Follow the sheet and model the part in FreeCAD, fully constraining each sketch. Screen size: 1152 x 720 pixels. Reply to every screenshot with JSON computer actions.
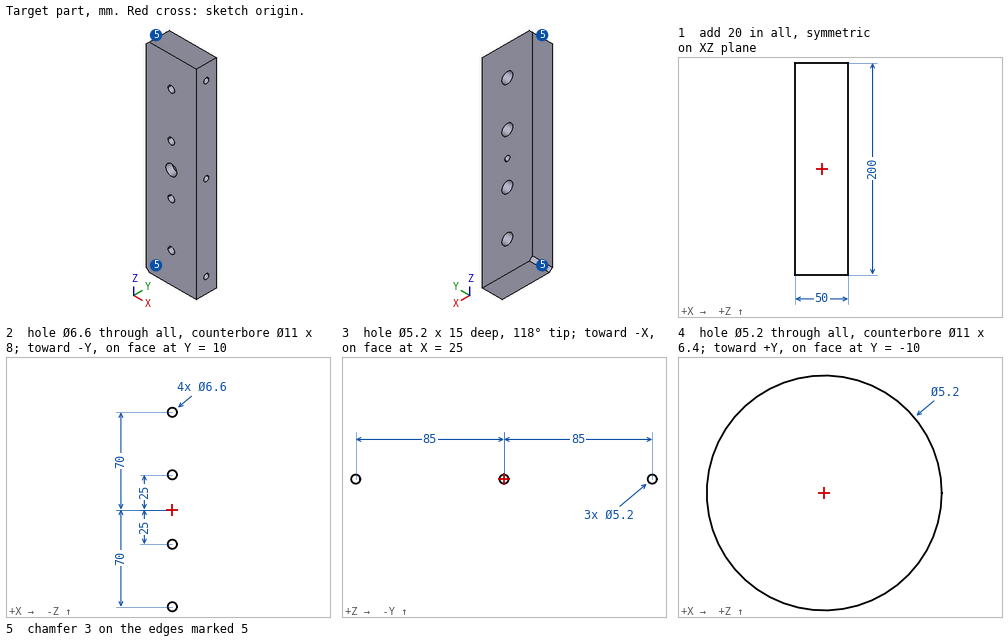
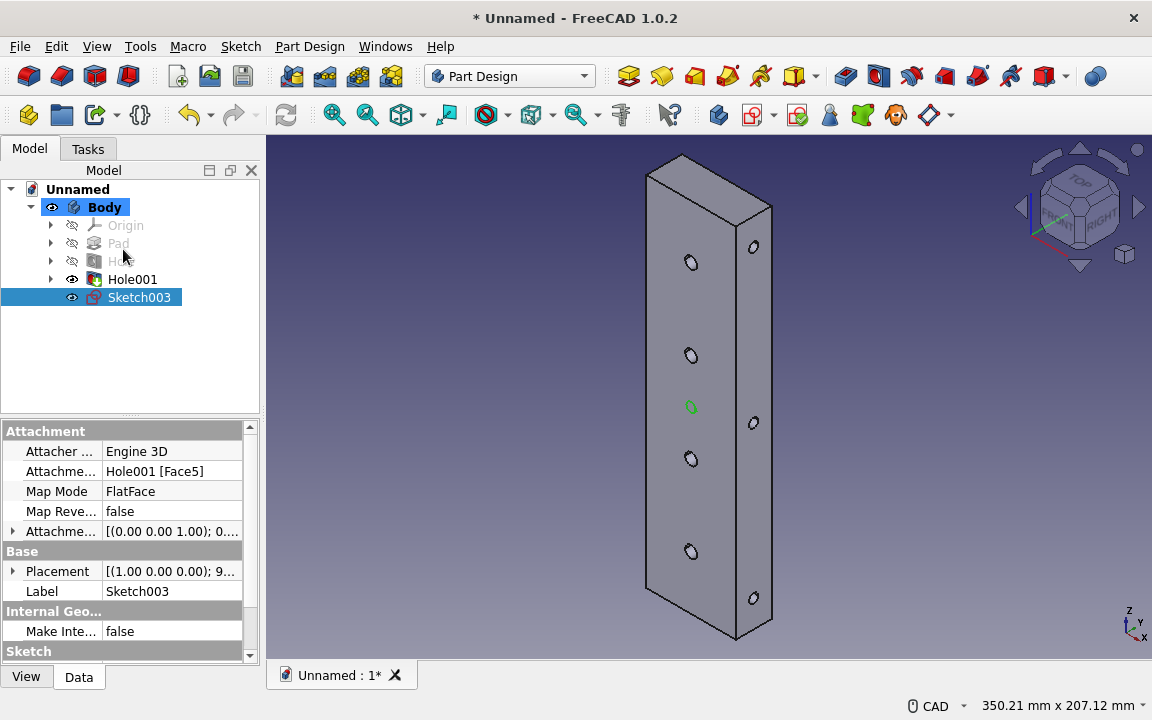
{"action": "left_click", "coordinate": [879, 76]}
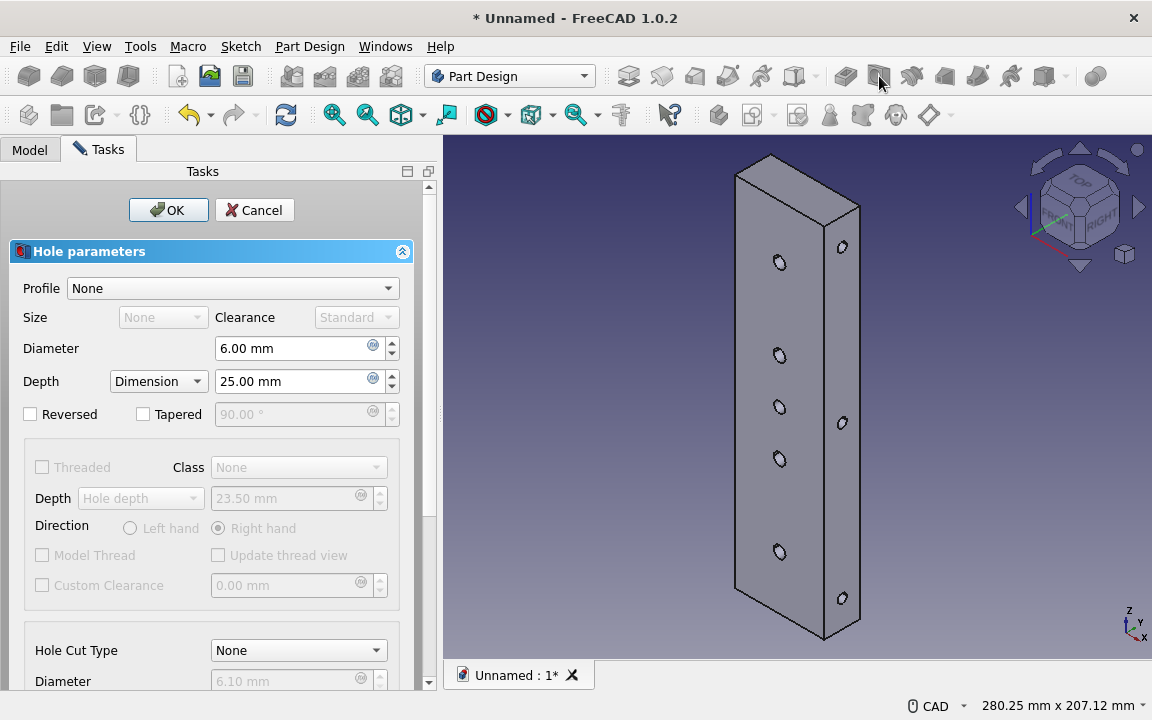
{"action": "triple_click", "coordinate": [300, 348]}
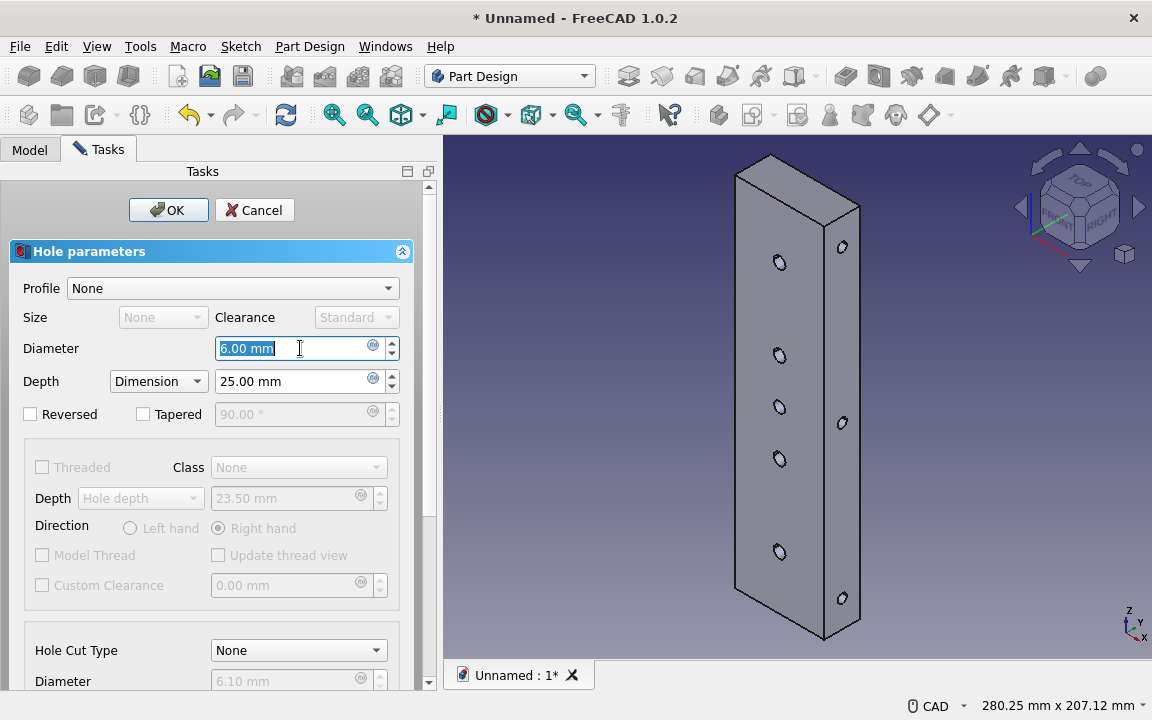
{"action": "type", "text": "5.2"}
{"action": "key", "text": "Tab"}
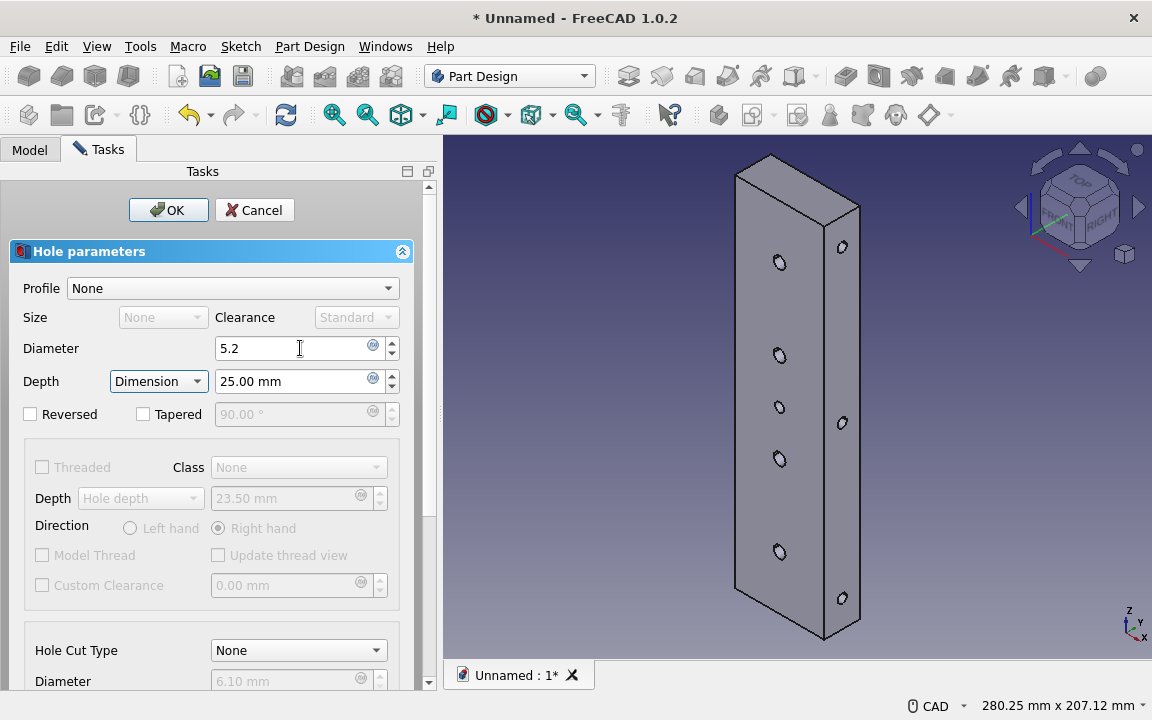
{"action": "left_click", "coordinate": [160, 382]}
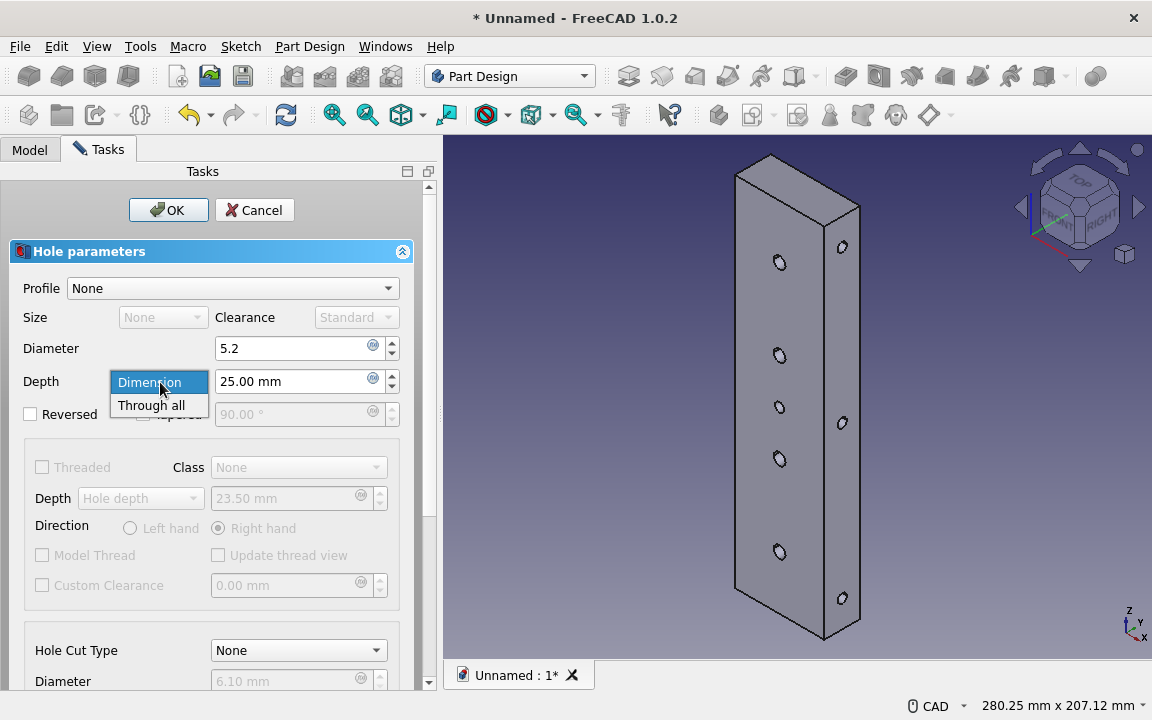
{"action": "left_click", "coordinate": [158, 406]}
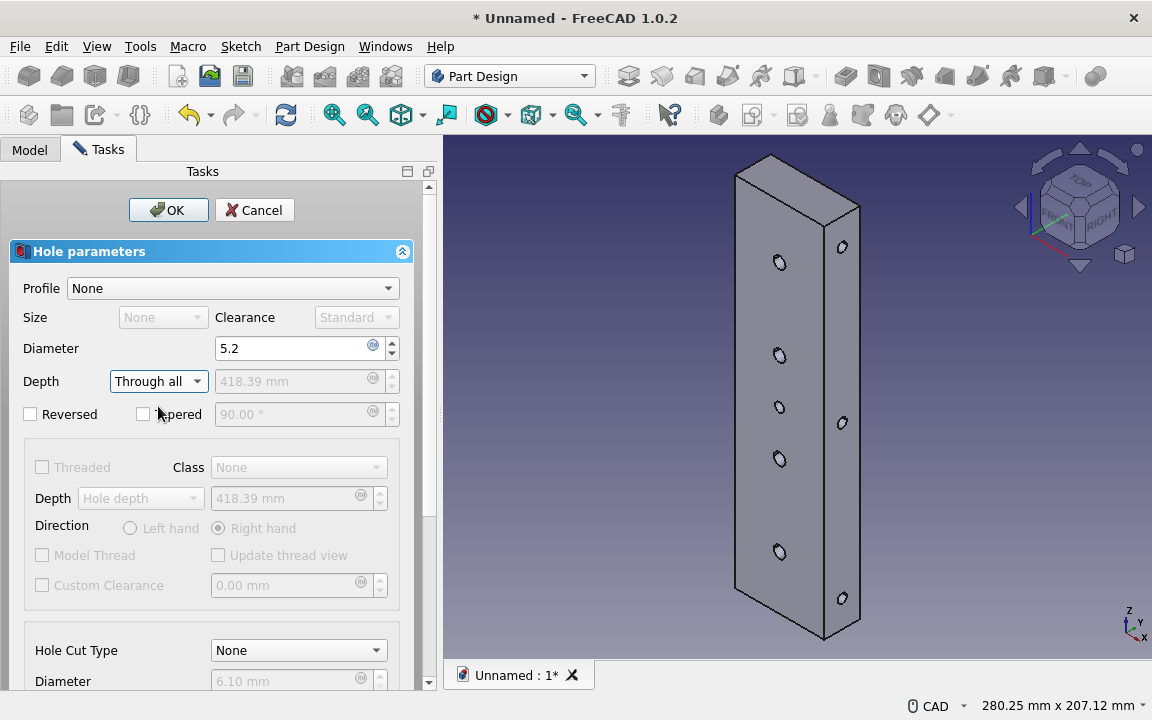
{"action": "left_click", "coordinate": [300, 650]}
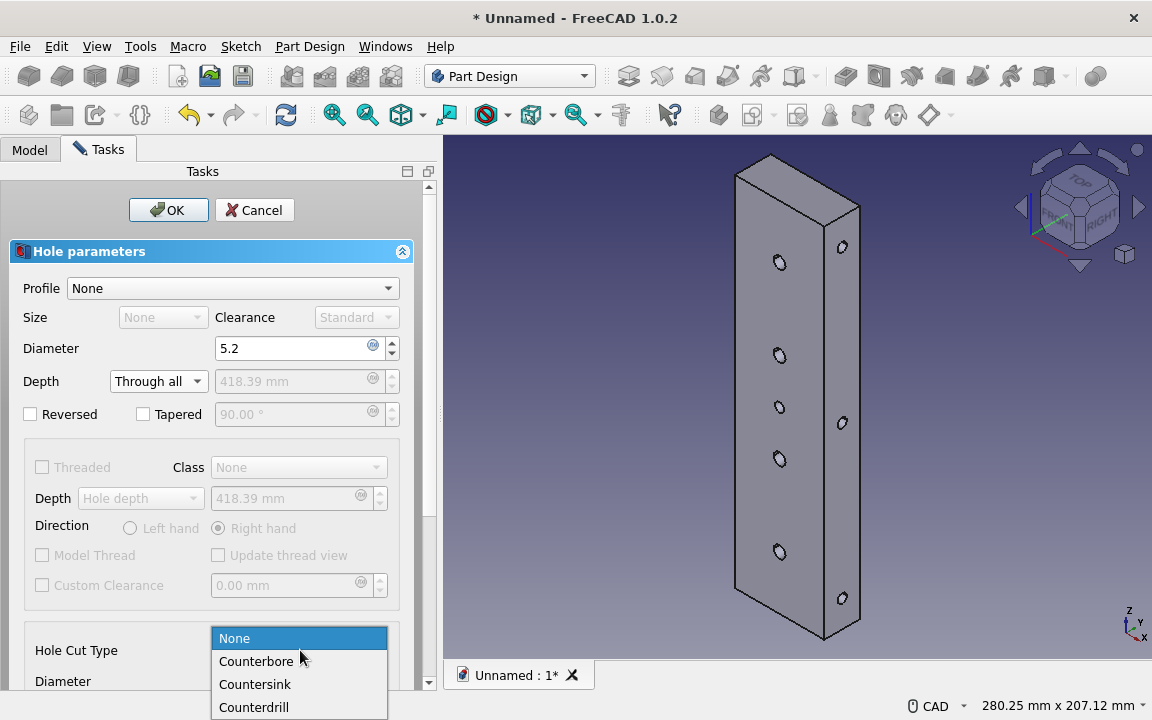
{"action": "left_click", "coordinate": [298, 662]}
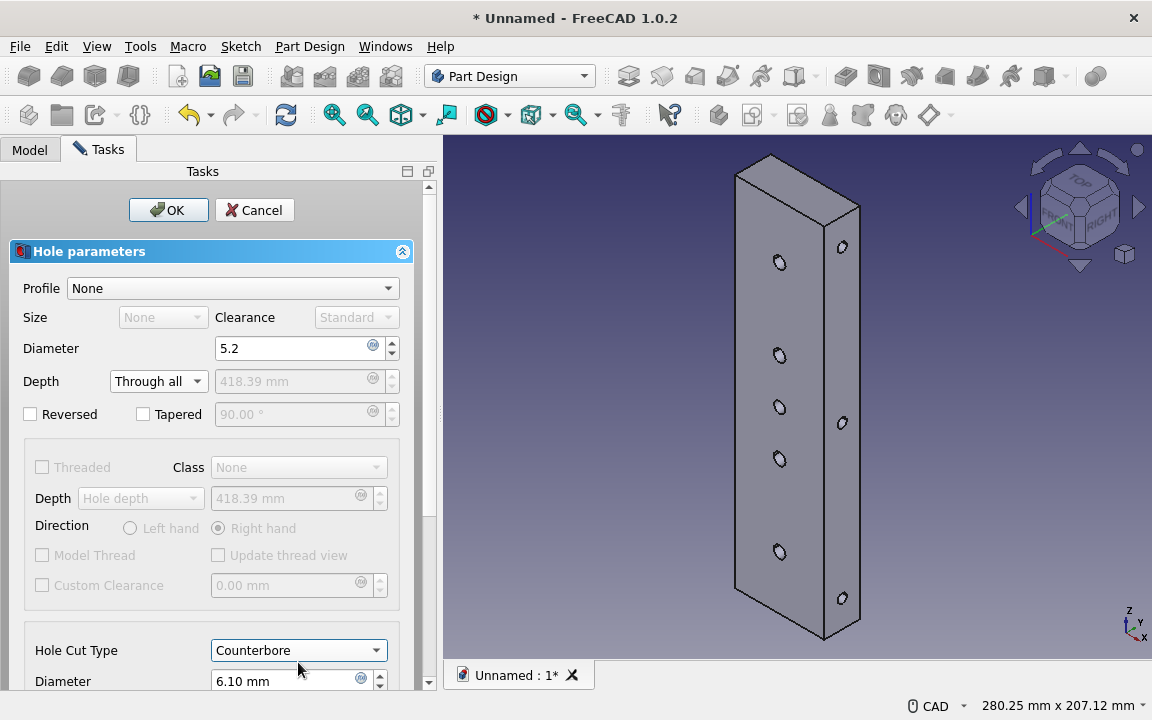
{"action": "scroll", "coordinate": [429, 436], "scroll_direction": "down", "scroll_amount": 2}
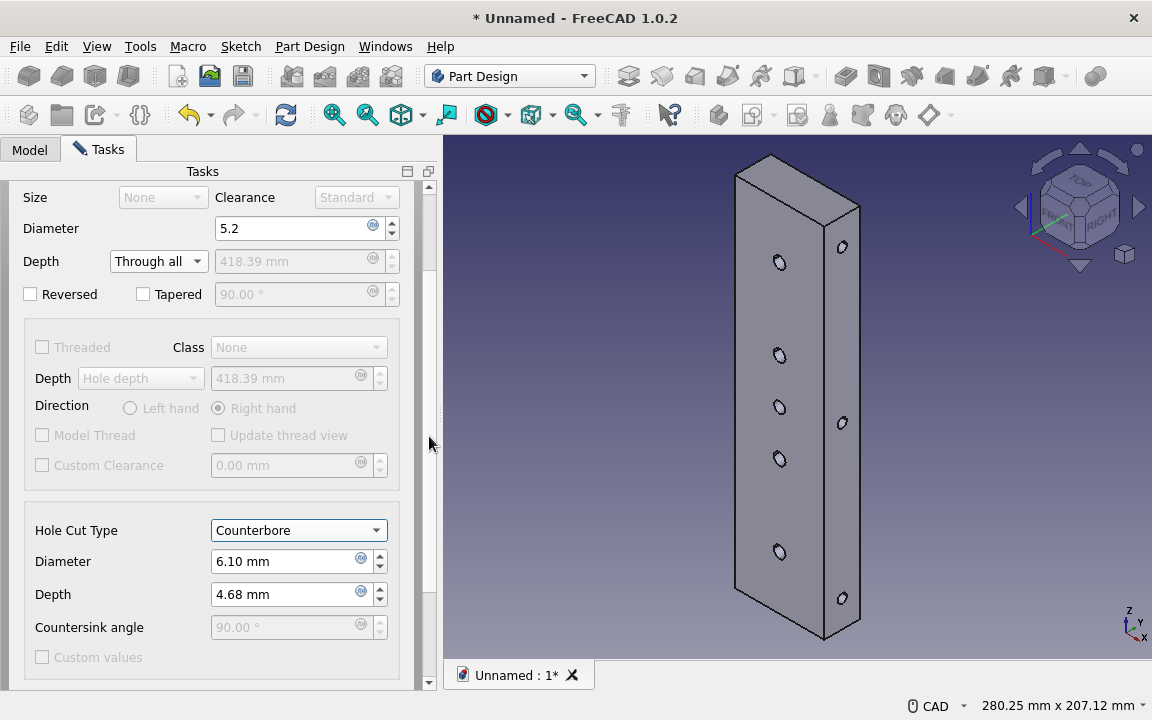
{"action": "triple_click", "coordinate": [292, 562]}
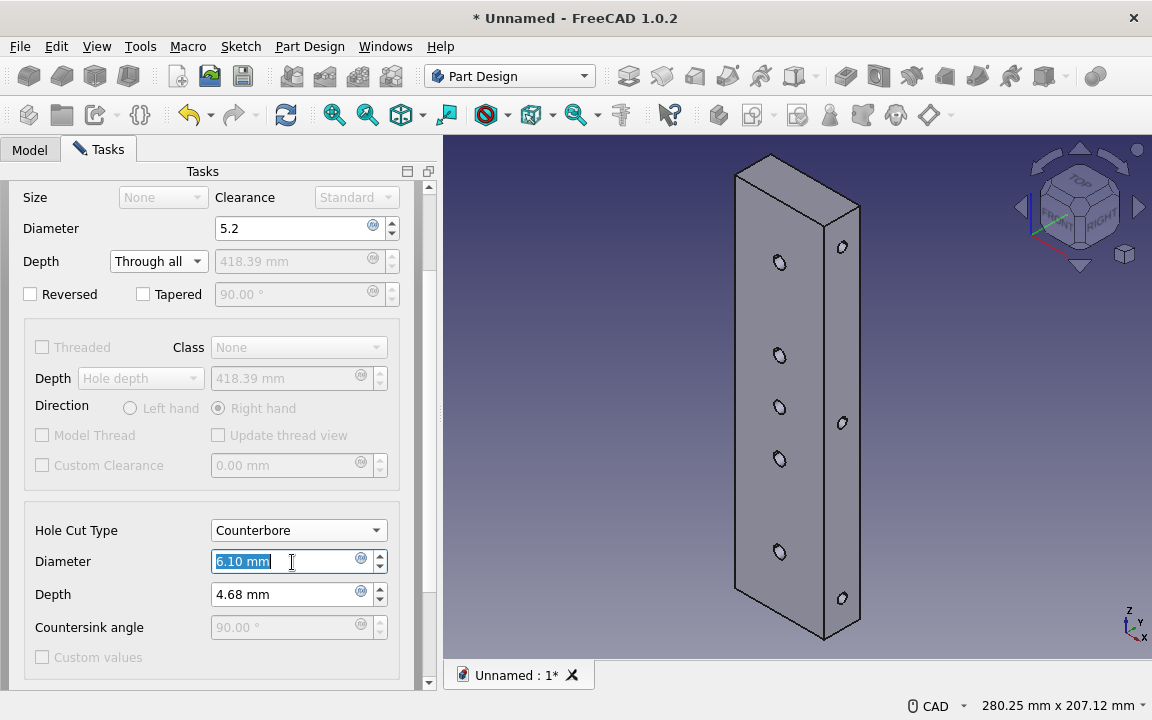
{"action": "type", "text": "11"}
{"action": "key", "text": "Tab"}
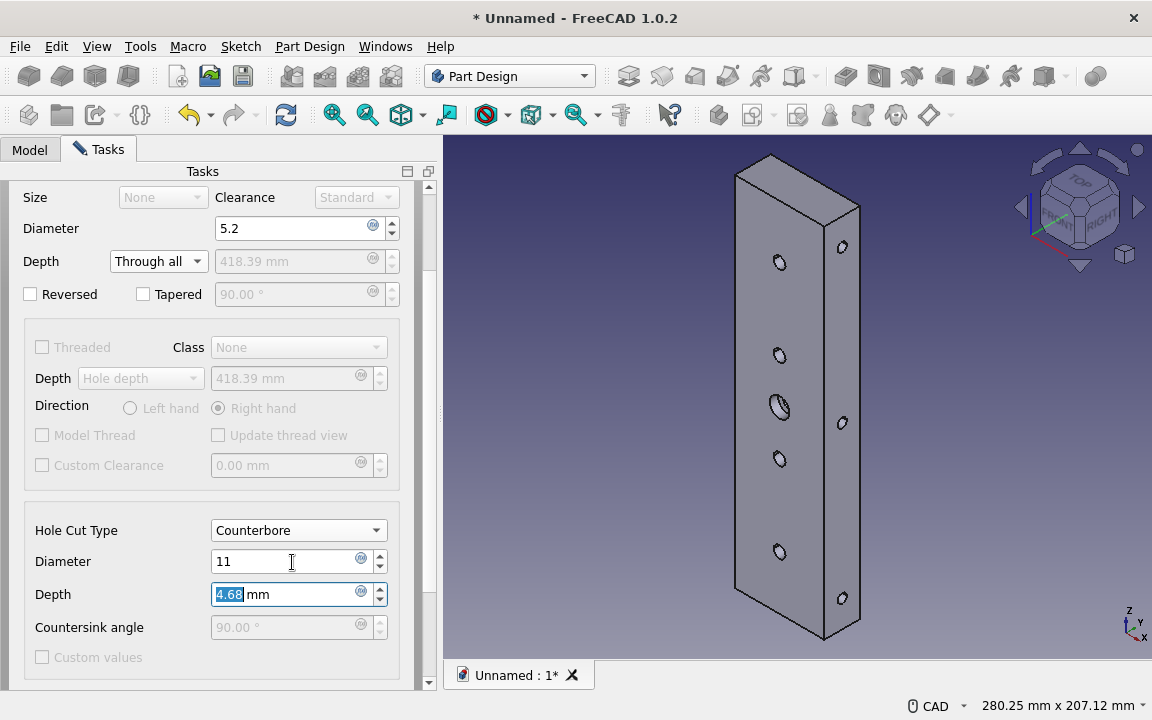
{"action": "type", "text": "6.4"}
{"action": "key", "text": "Tab"}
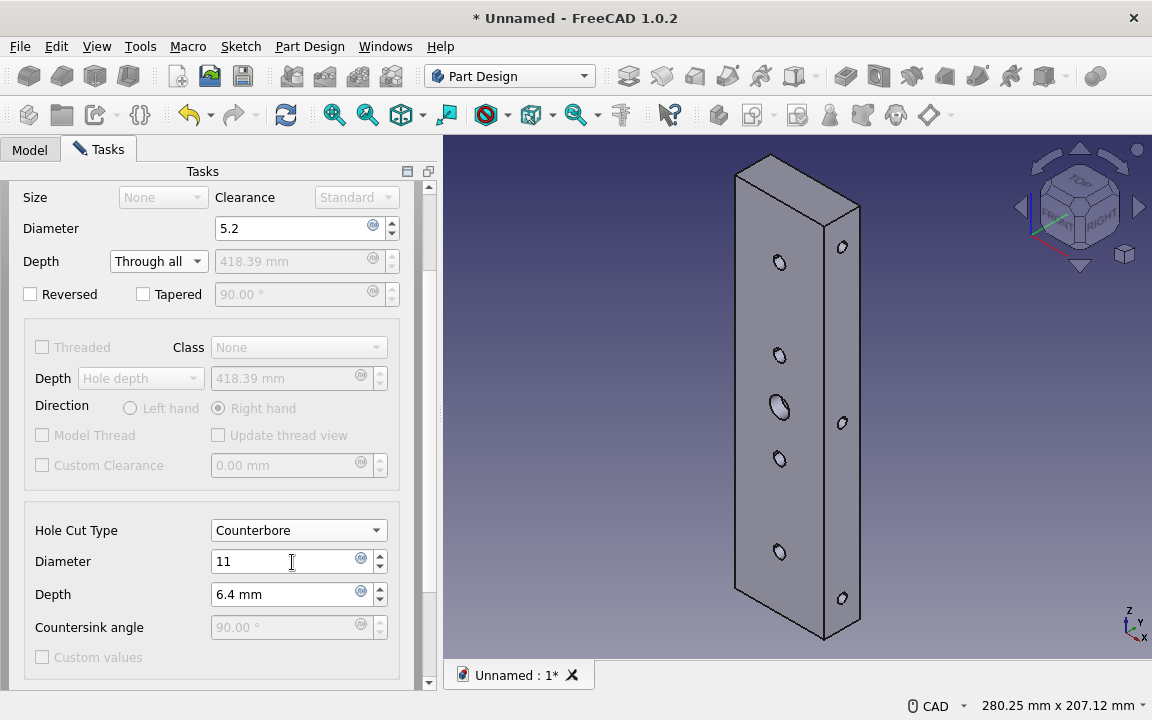
{"action": "scroll", "coordinate": [429, 436], "scroll_direction": "up", "scroll_amount": 3}